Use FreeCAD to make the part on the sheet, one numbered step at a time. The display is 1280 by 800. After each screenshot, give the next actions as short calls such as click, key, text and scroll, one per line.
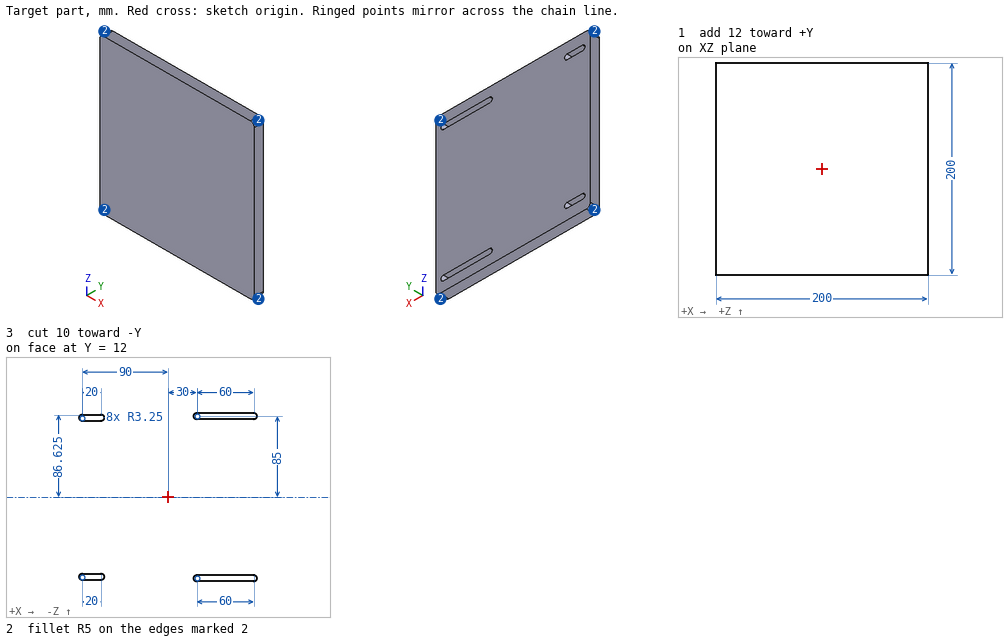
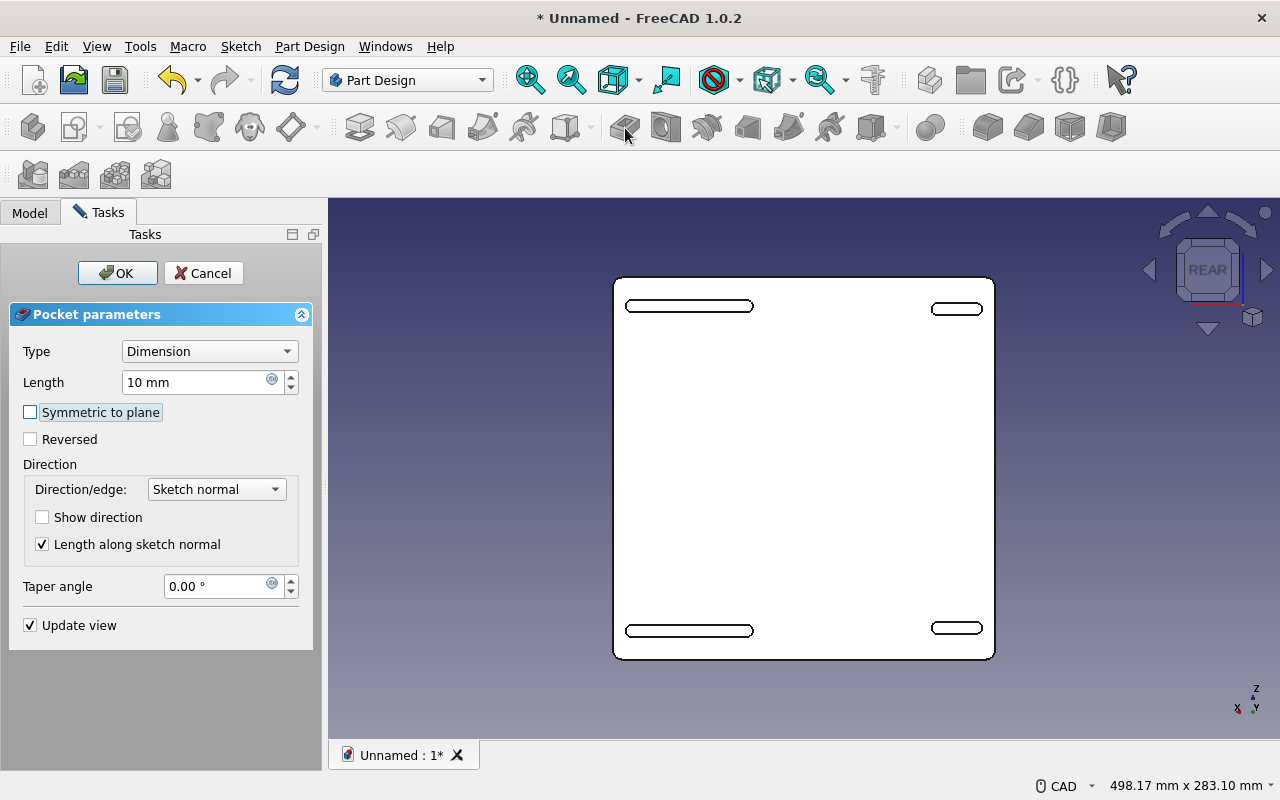
click(118, 273)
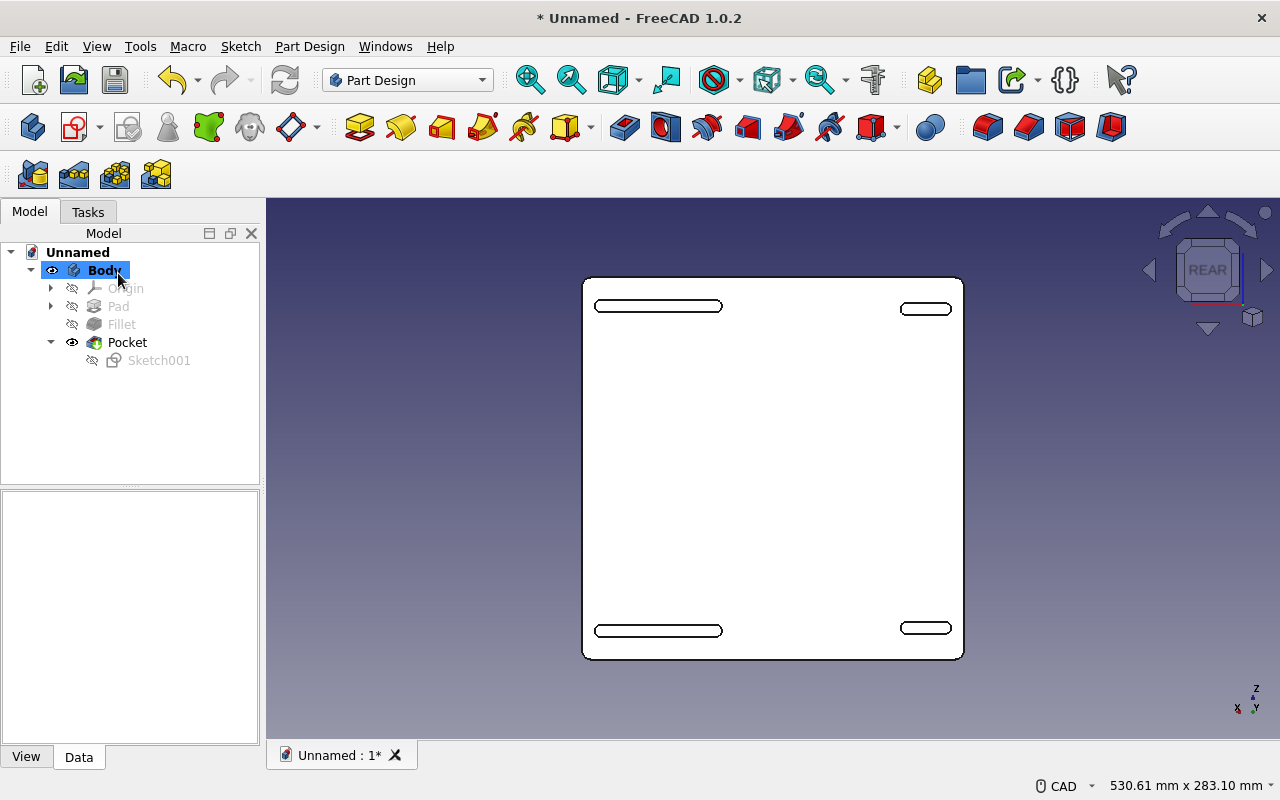
key(0)